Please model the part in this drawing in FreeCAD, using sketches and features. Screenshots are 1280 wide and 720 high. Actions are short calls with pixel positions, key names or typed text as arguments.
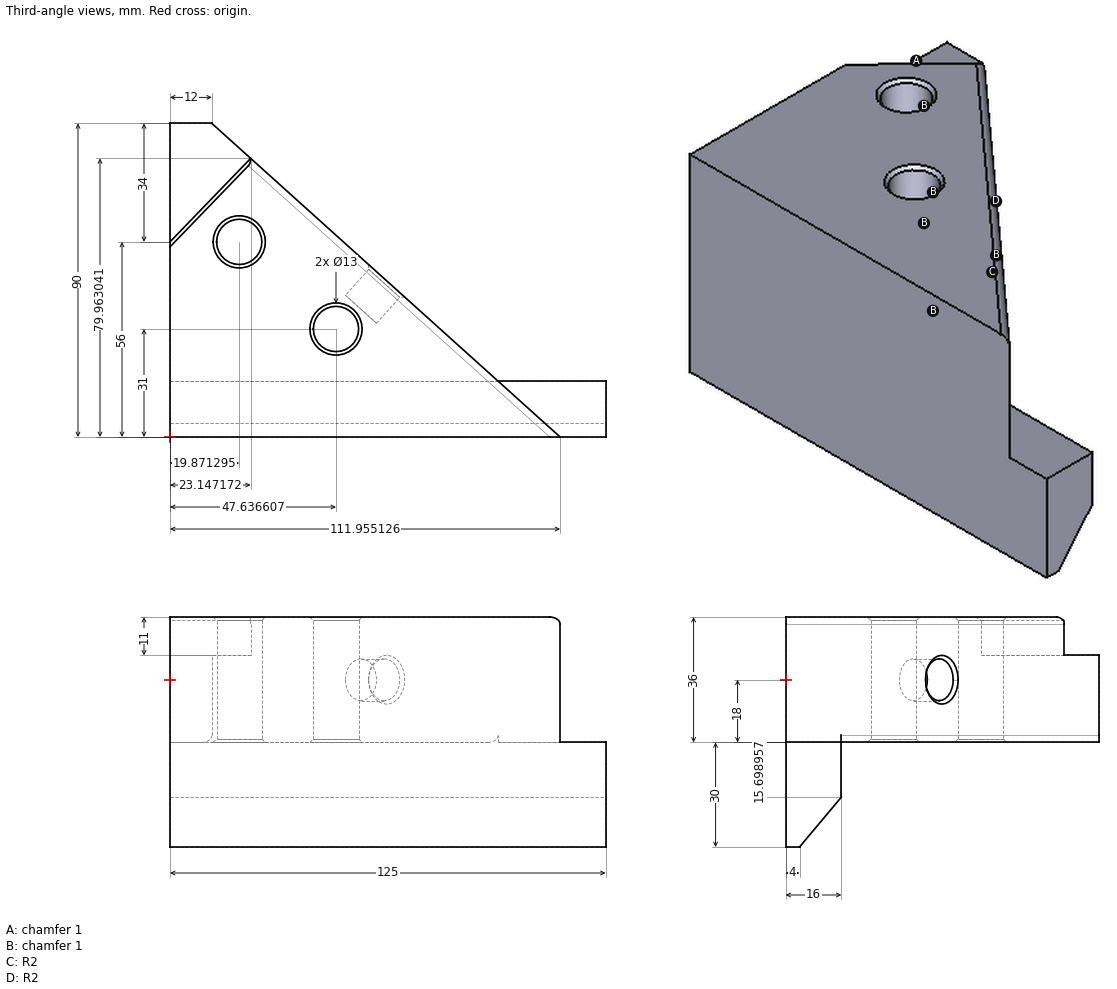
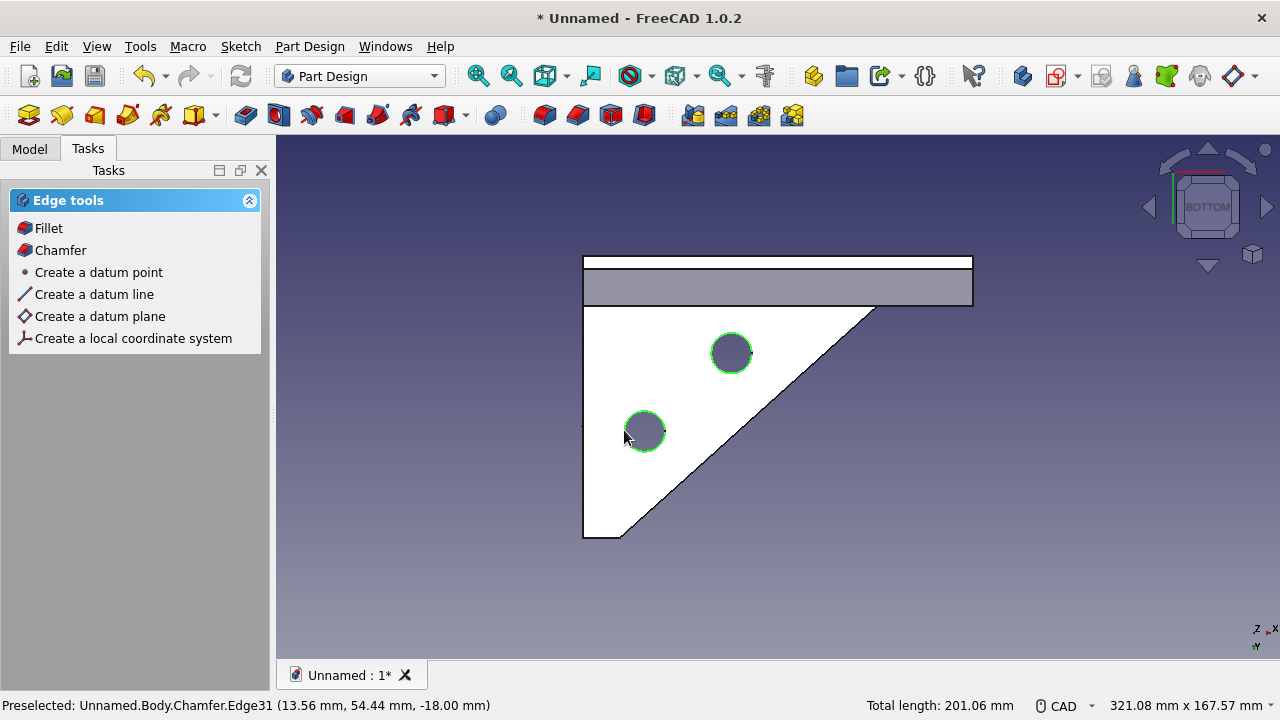
click(578, 116)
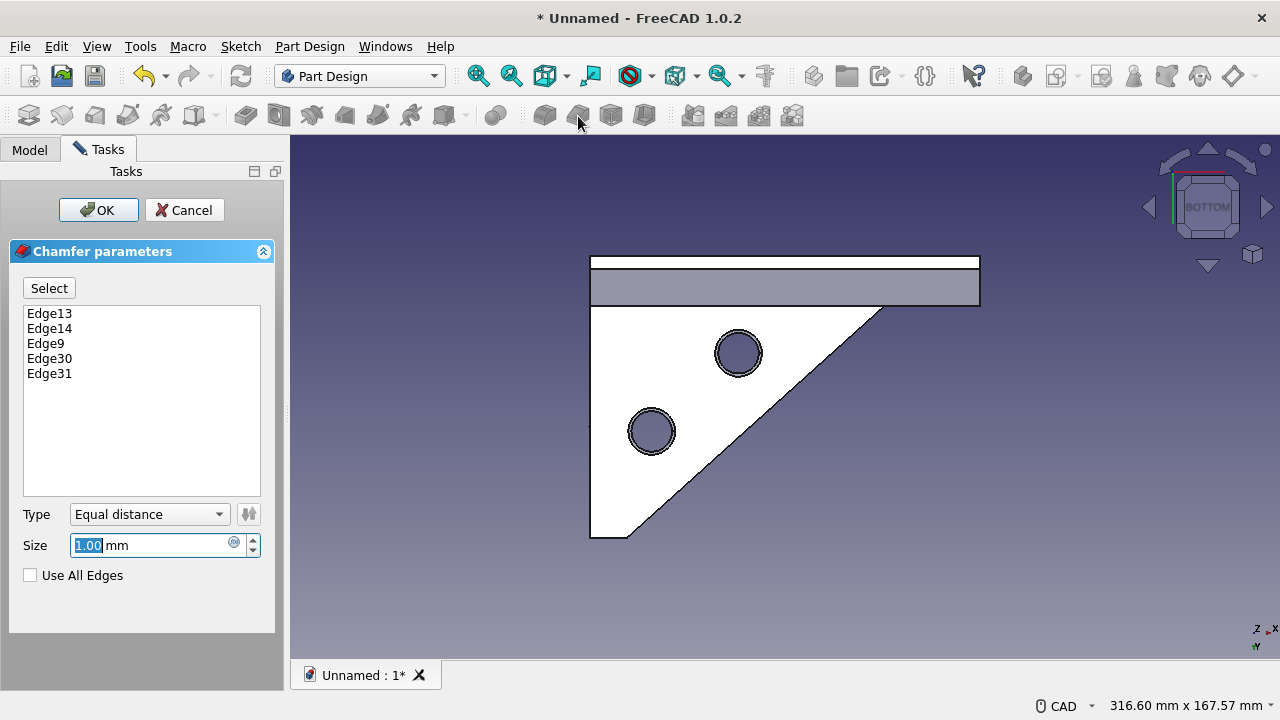
text(1)
key(Tab)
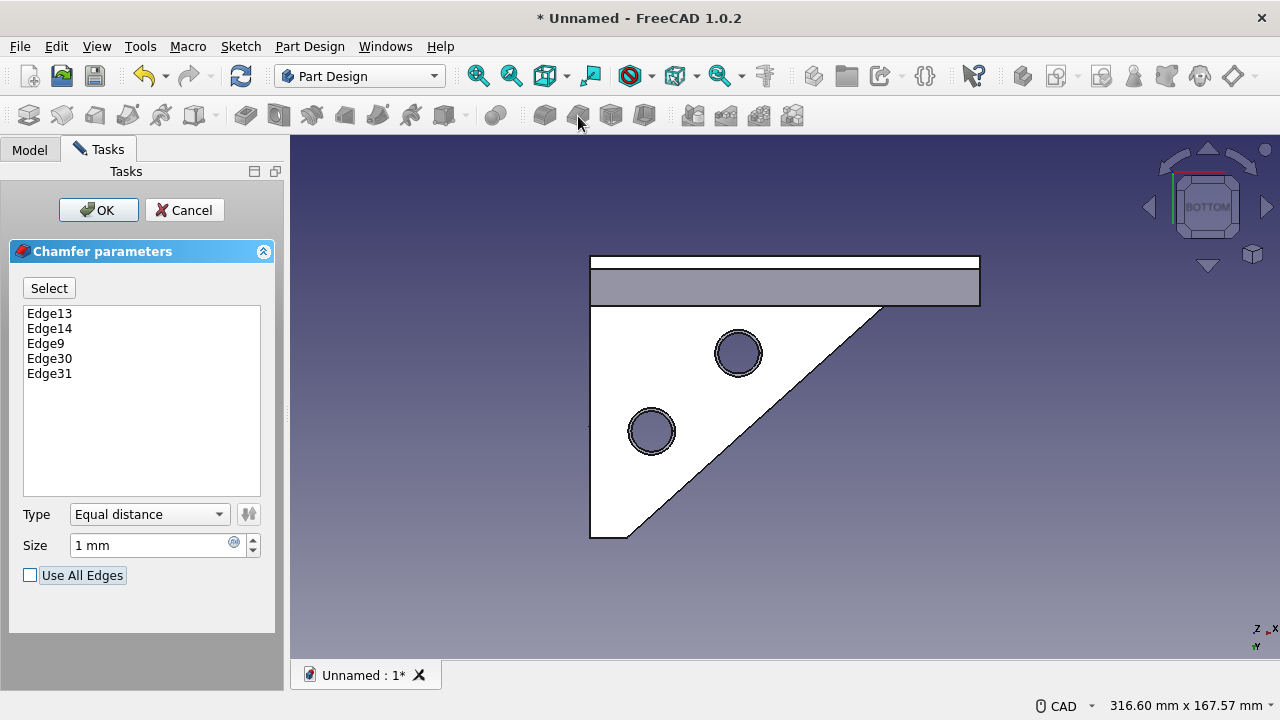
click(99, 210)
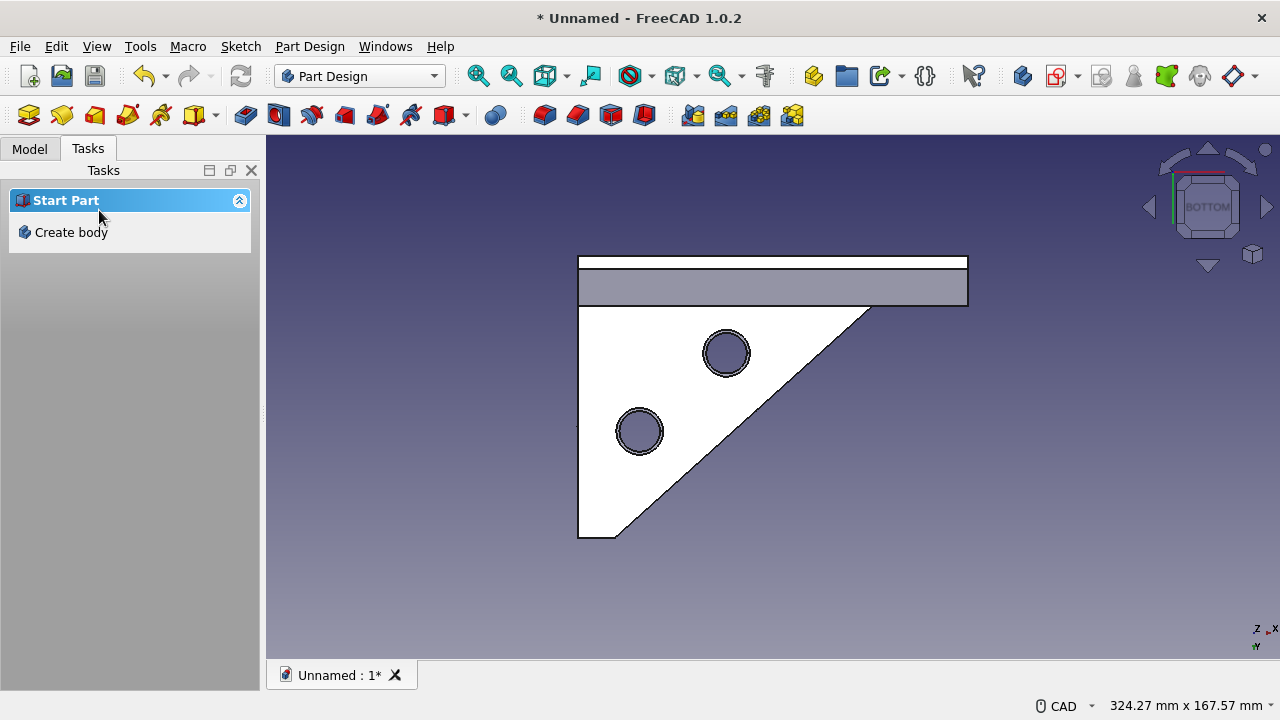
click(744, 421)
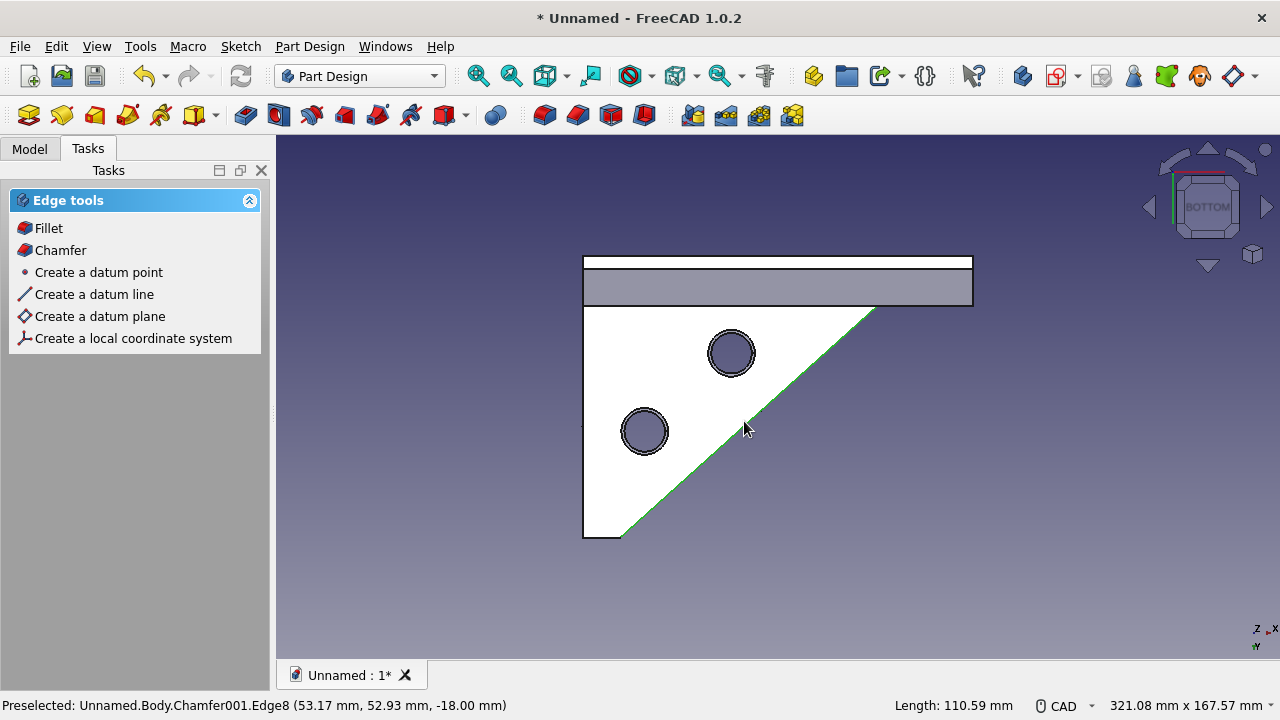
click(545, 116)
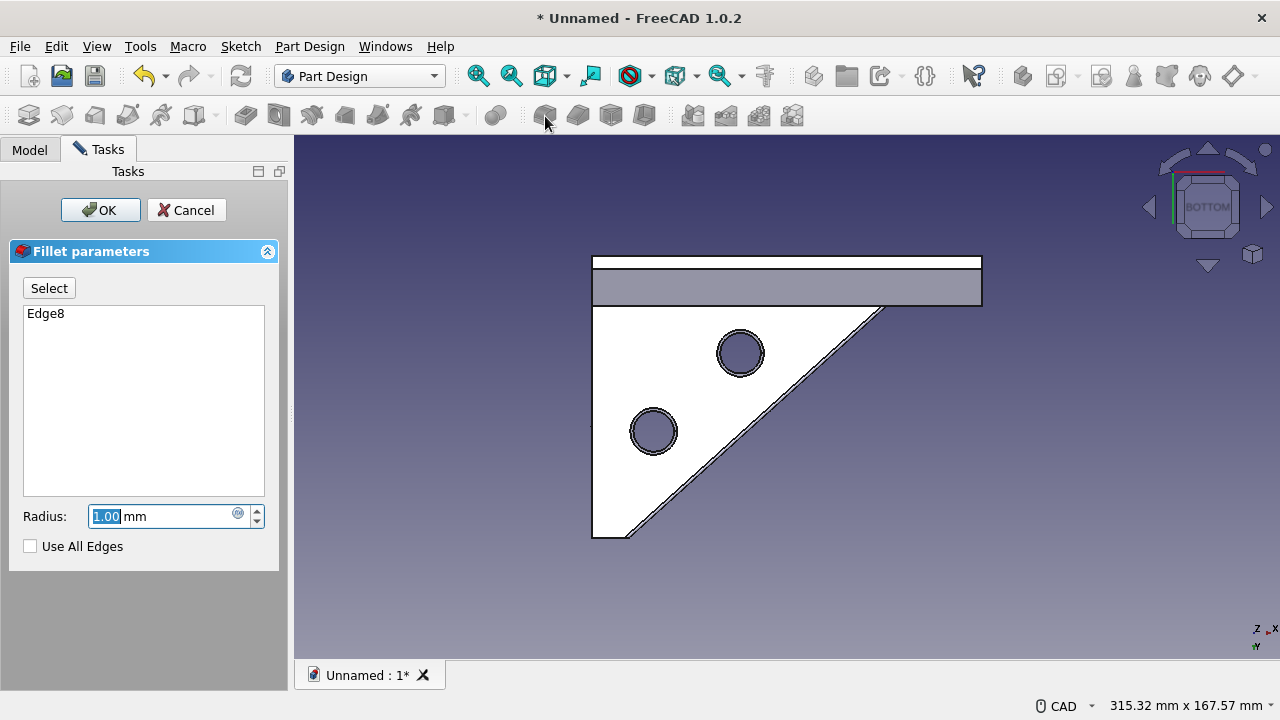
text(2)
key(Tab)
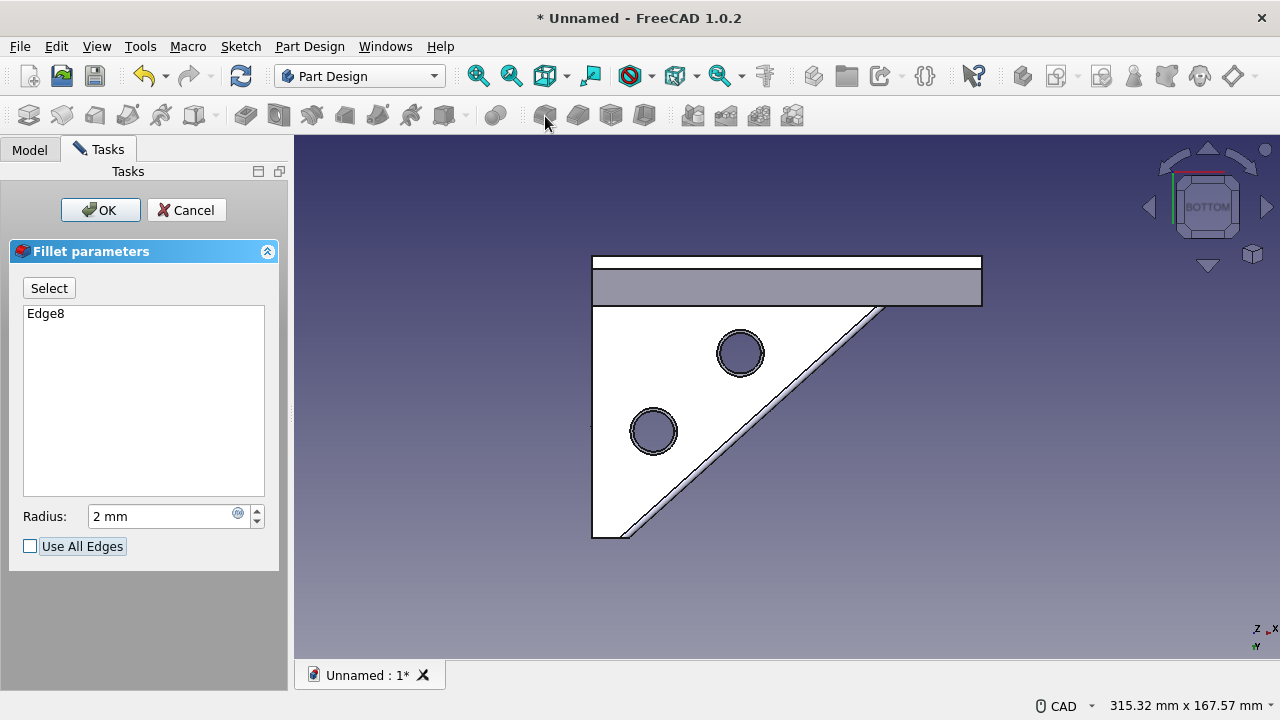
click(101, 210)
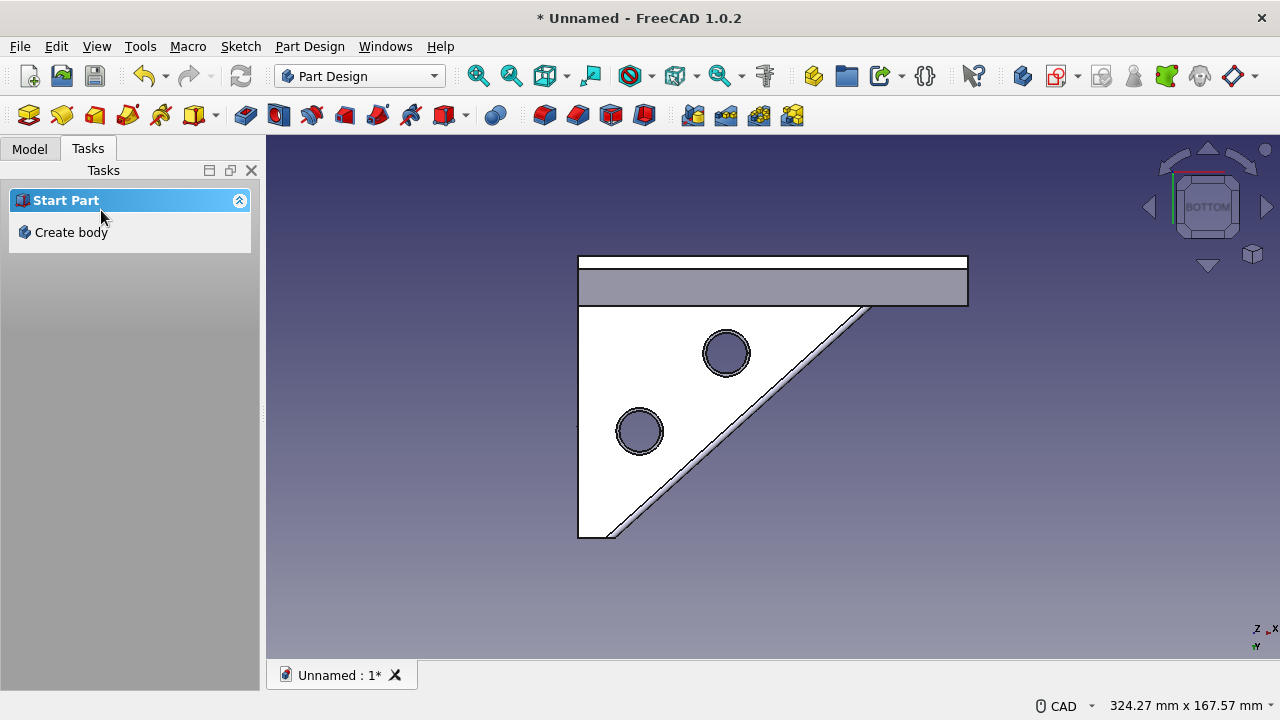
key(0)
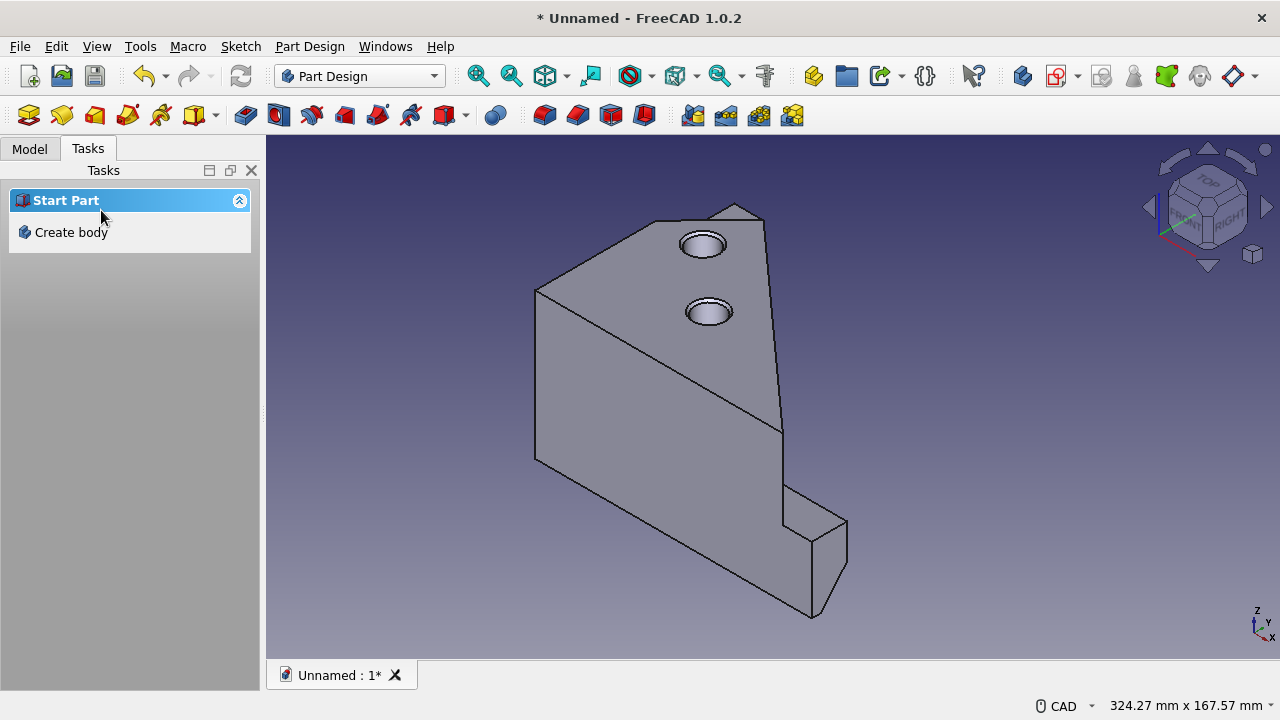
key(2)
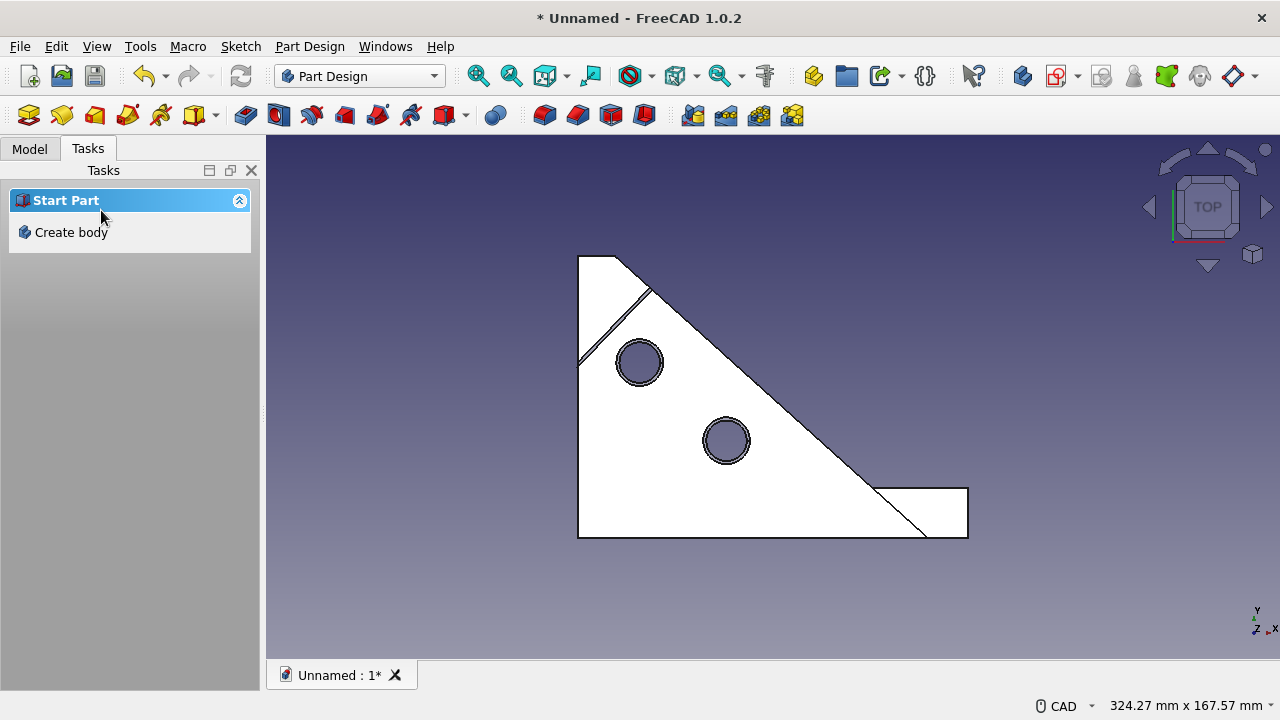
click(790, 413)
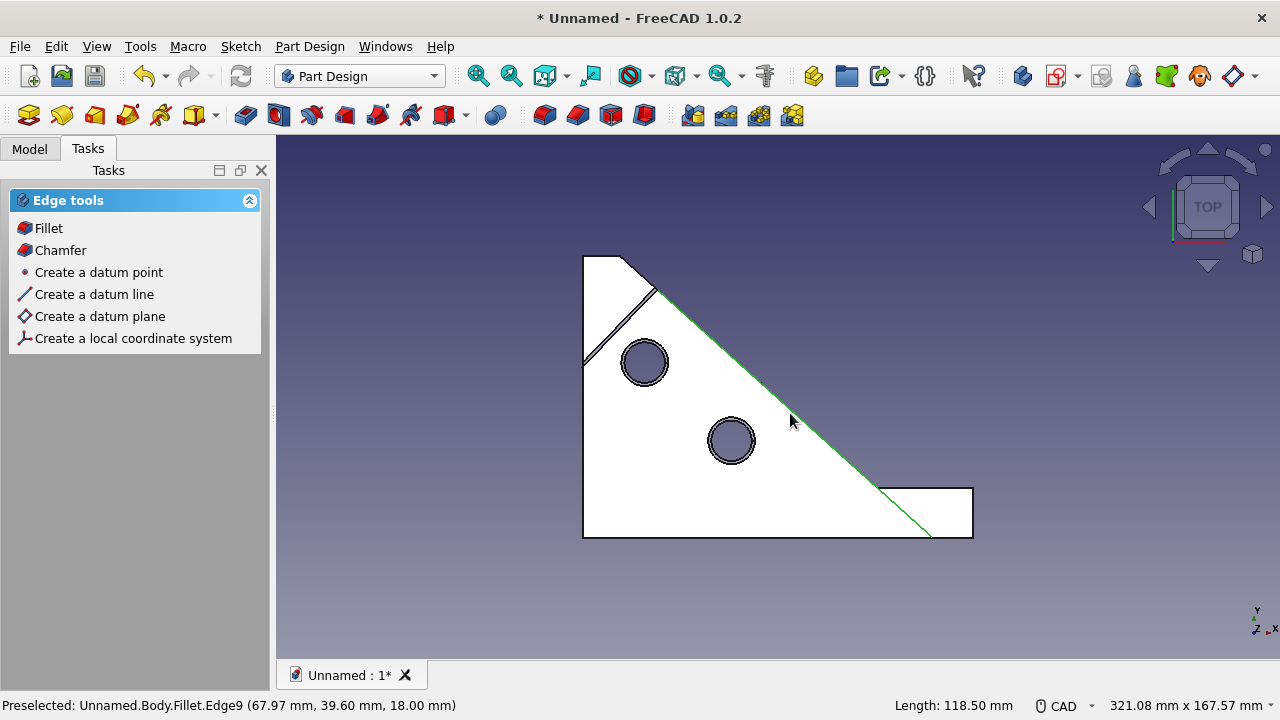
click(545, 116)